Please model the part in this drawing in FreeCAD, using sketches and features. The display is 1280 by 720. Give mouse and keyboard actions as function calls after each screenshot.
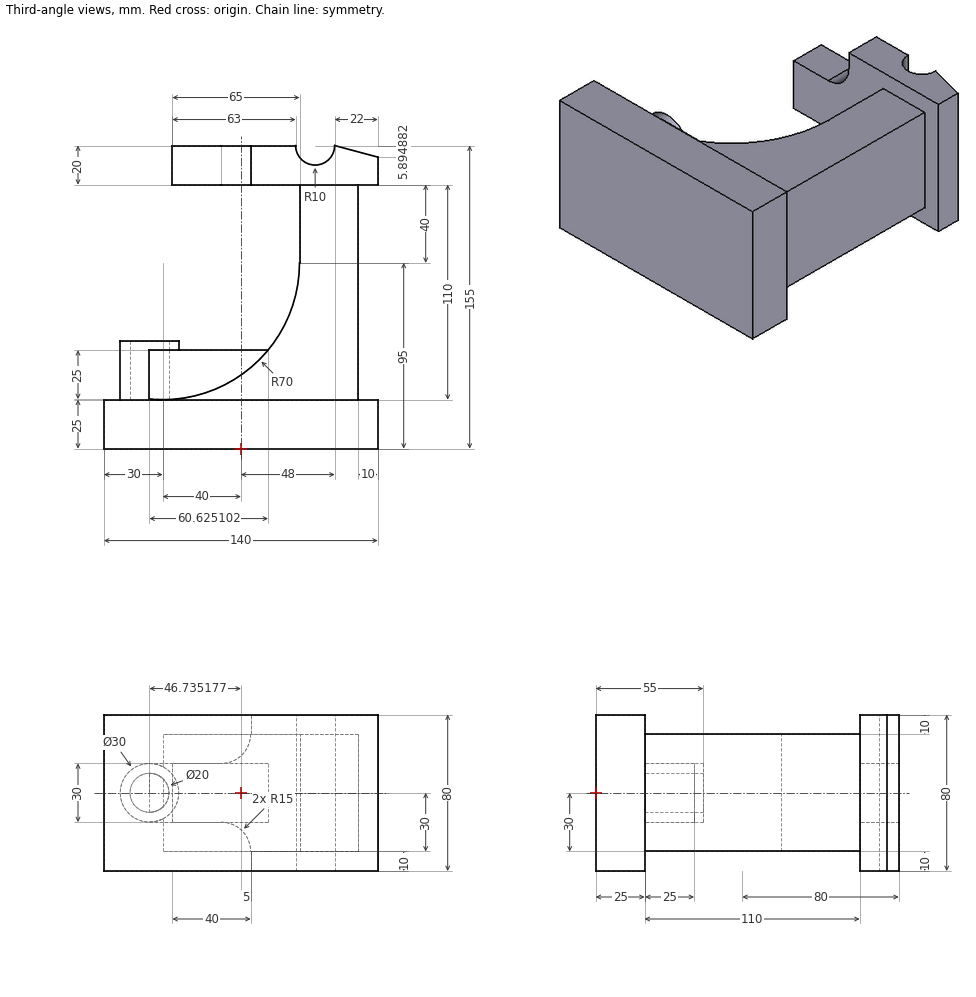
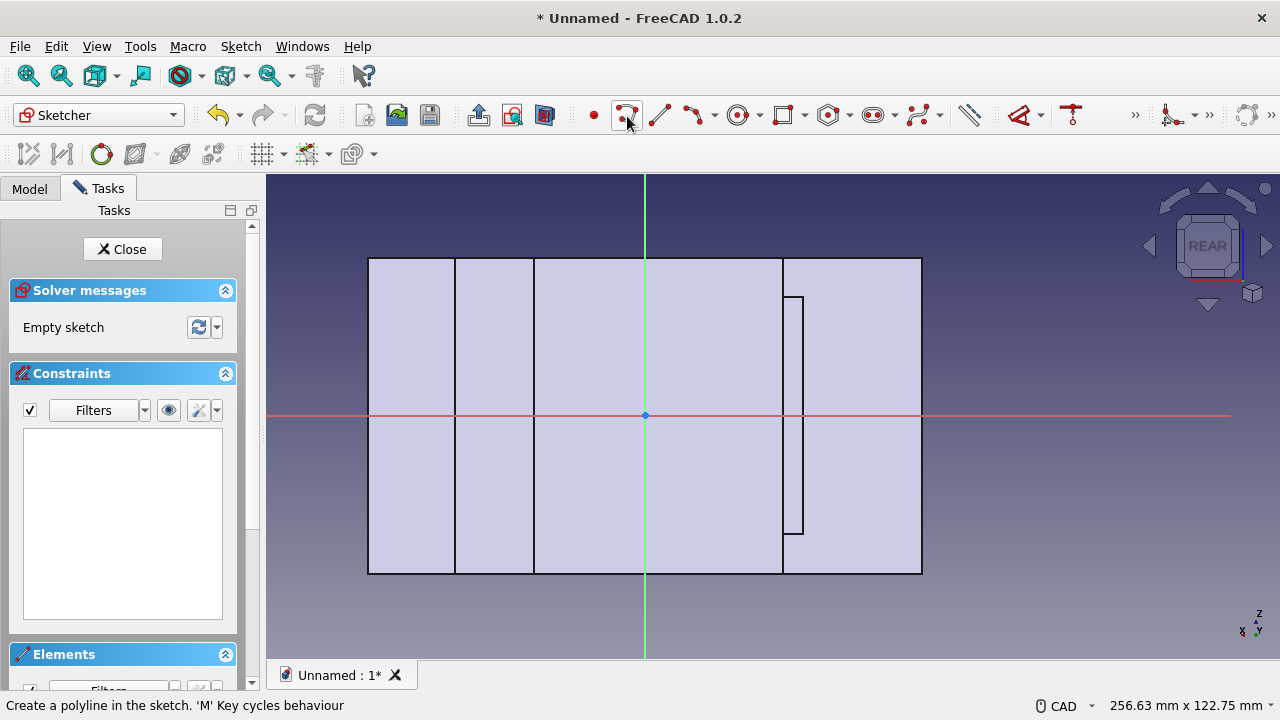
click(625, 534)
click(625, 574)
click(783, 574)
click(783, 475)
click(685, 475)
right_click(685, 475)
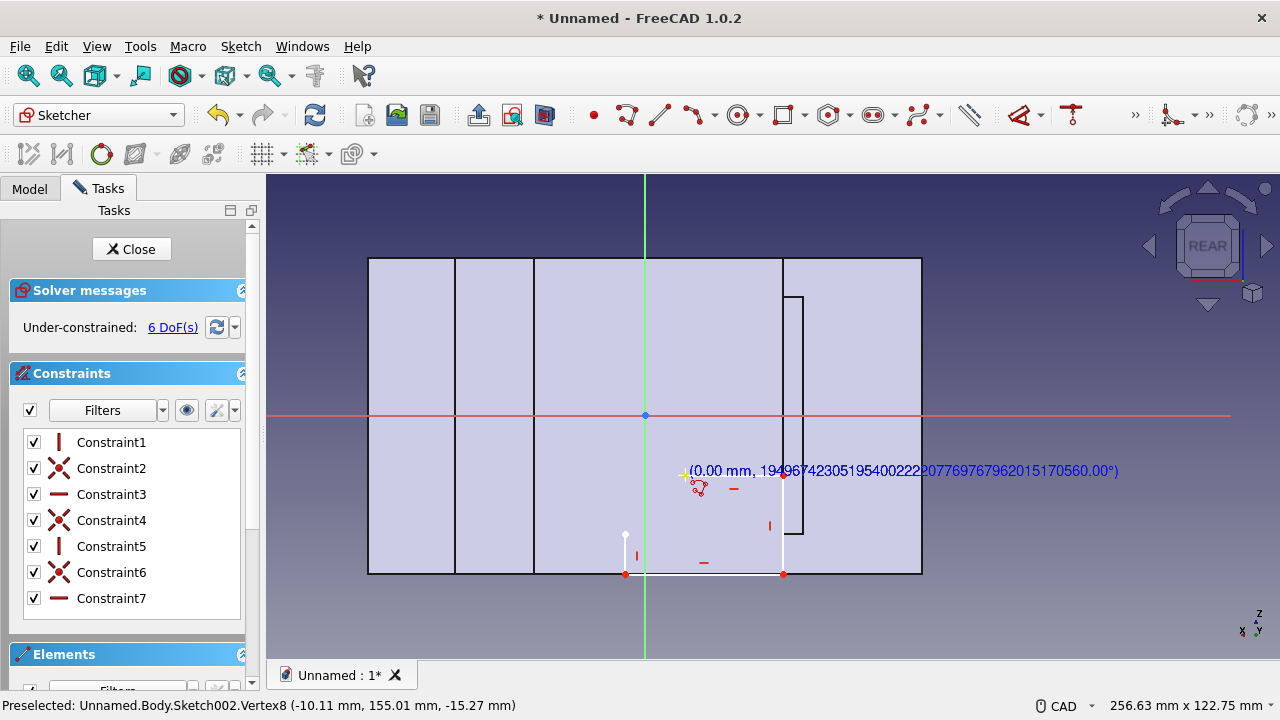
click(692, 116)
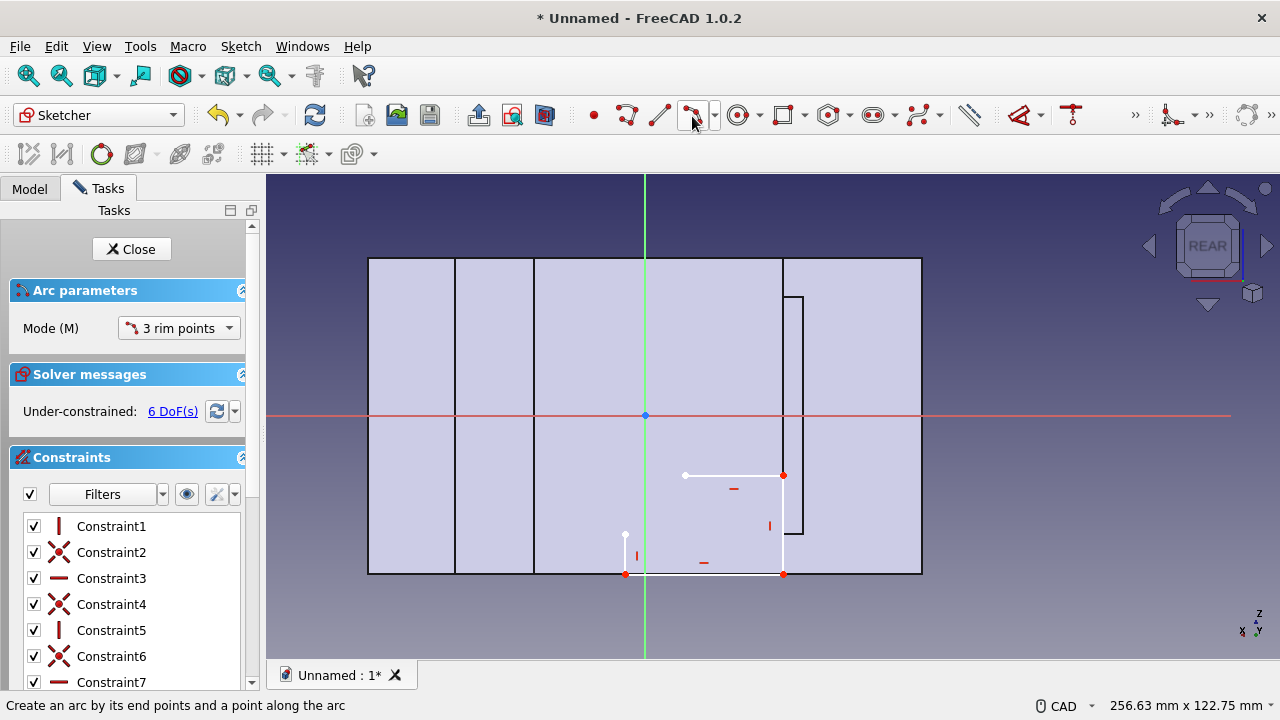
click(685, 476)
click(625, 535)
click(632, 507)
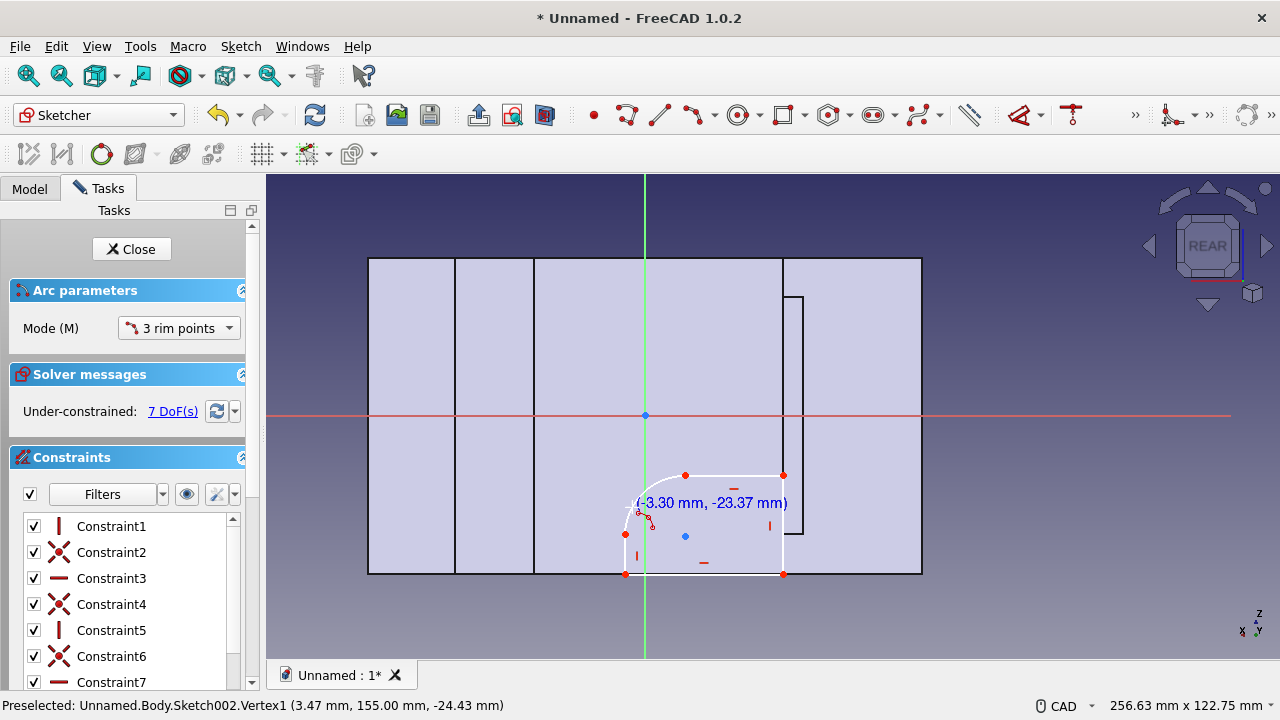
click(627, 116)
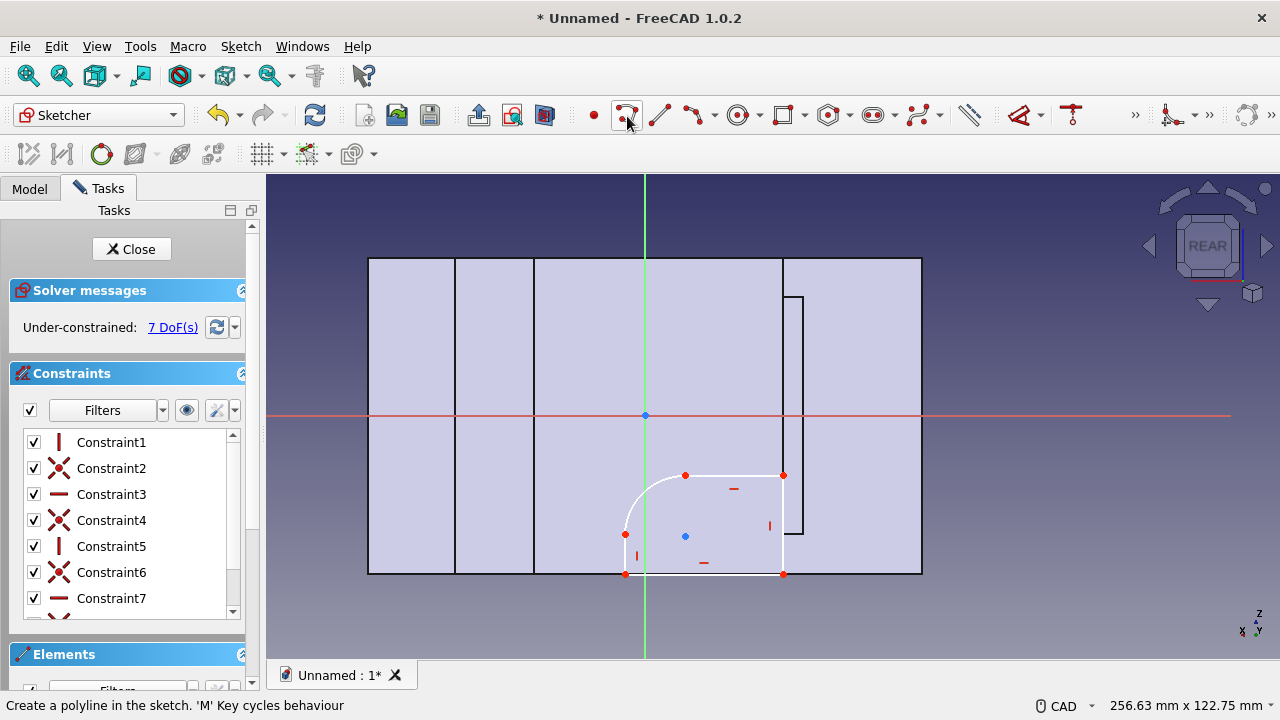
click(685, 356)
click(783, 356)
click(783, 258)
click(625, 258)
click(625, 297)
right_click(625, 297)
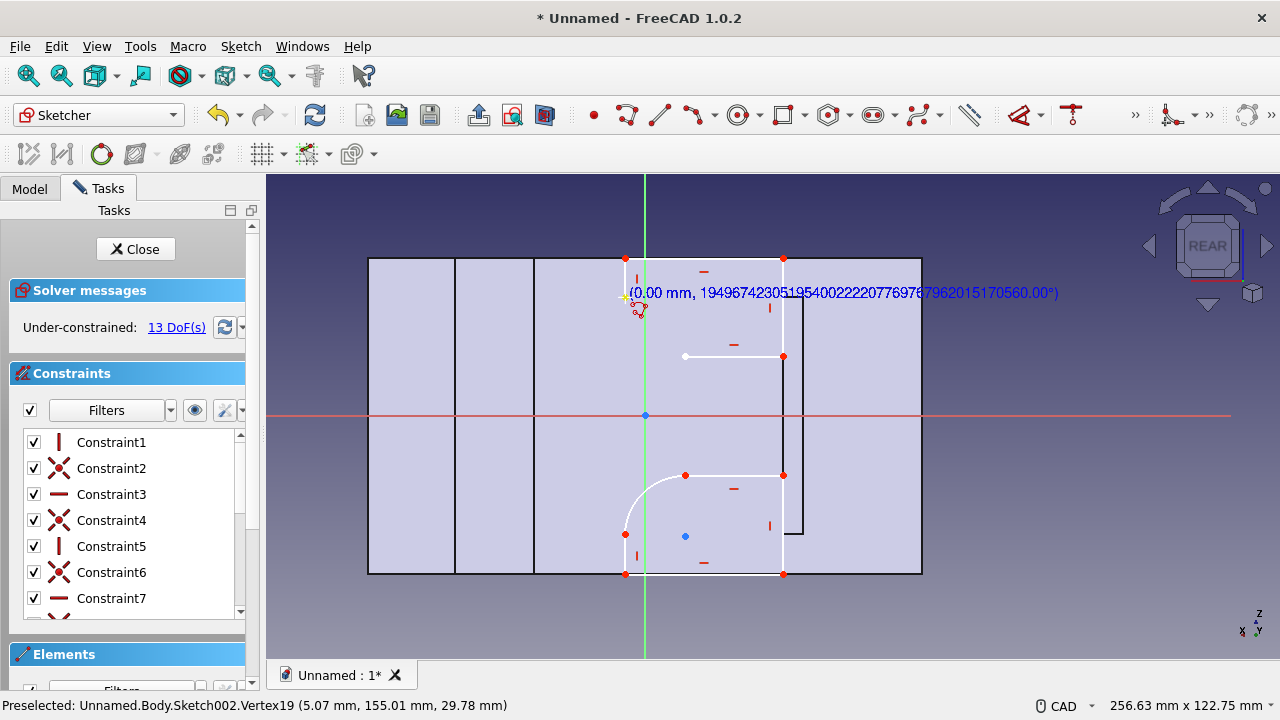
click(692, 116)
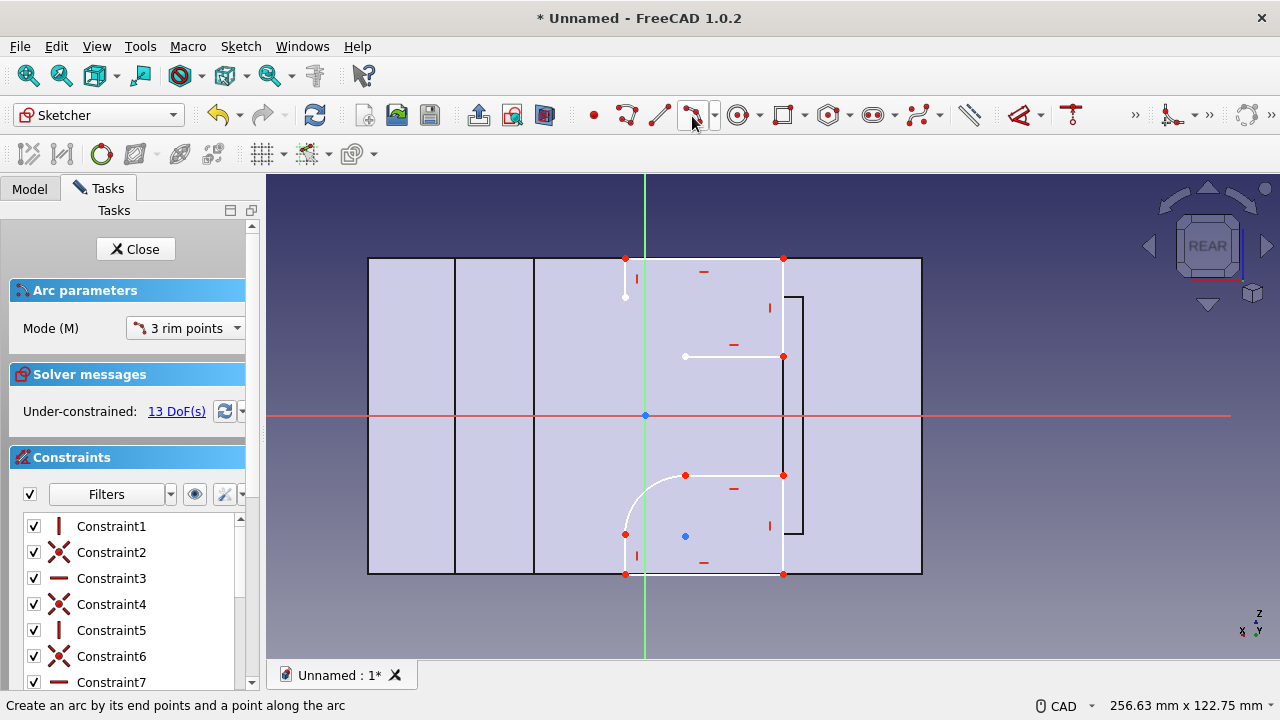
click(625, 298)
click(685, 357)
click(632, 324)
key(Escape)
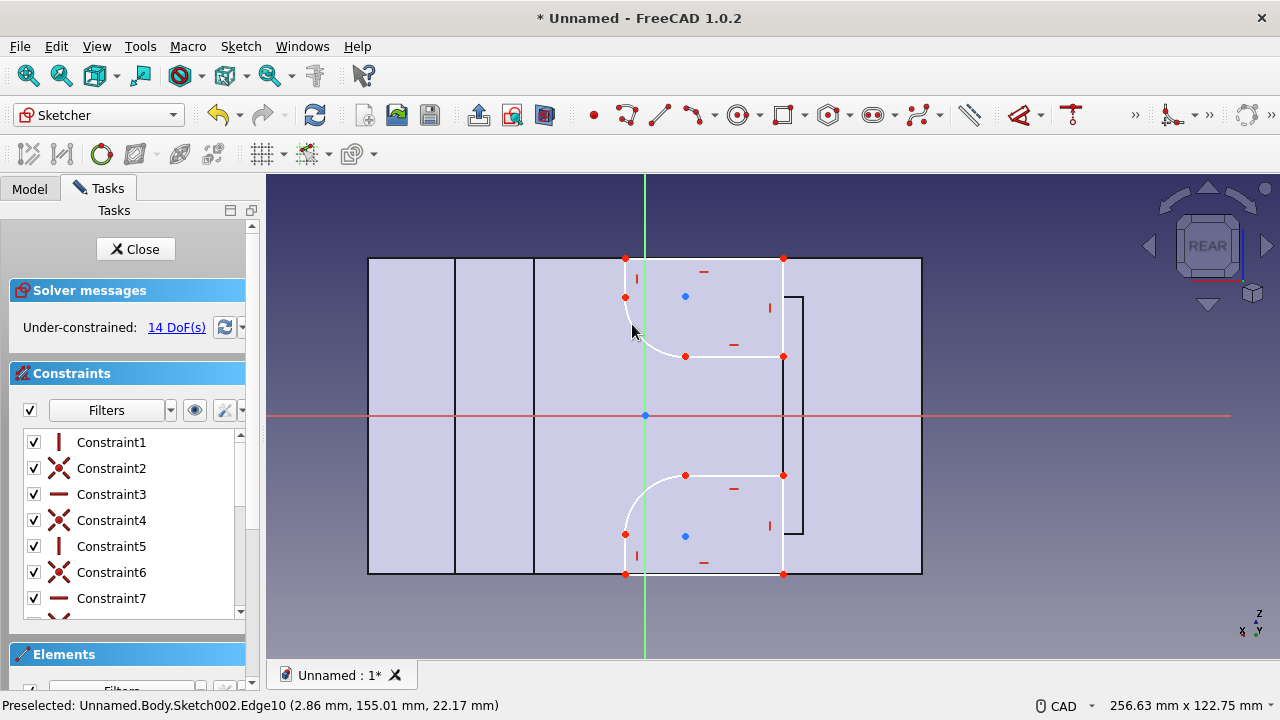
click(625, 547)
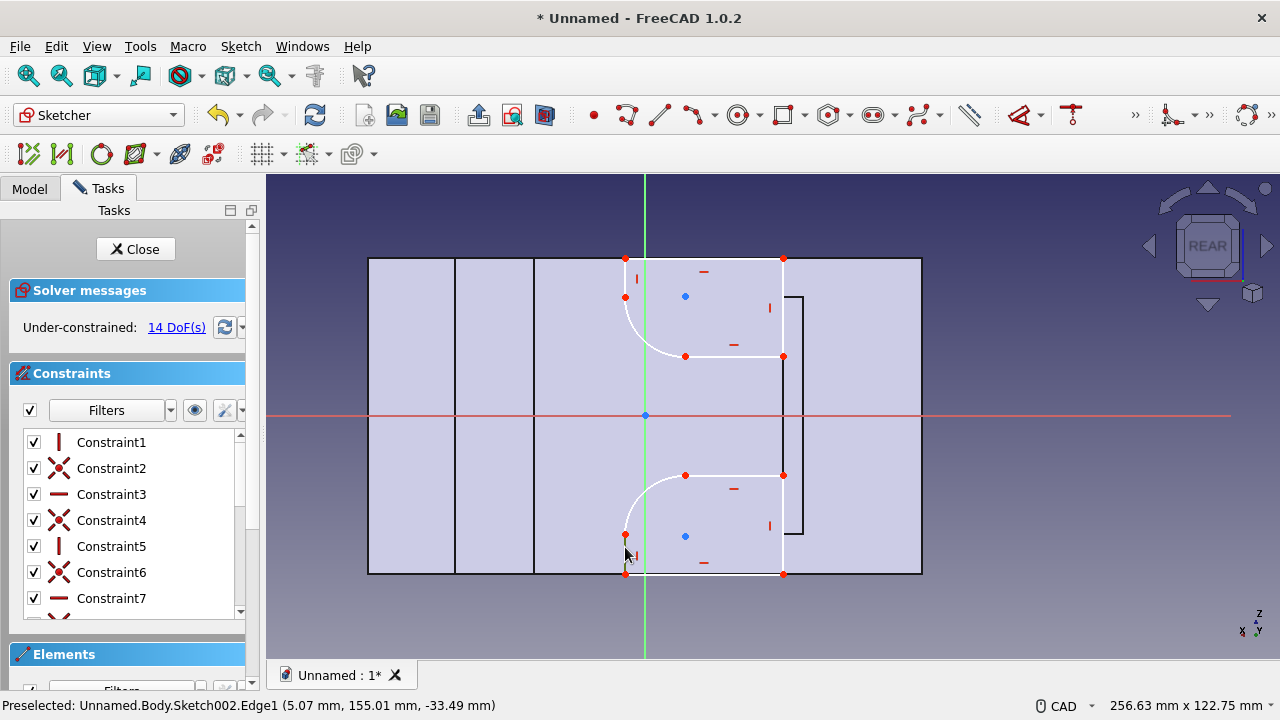
click(658, 482)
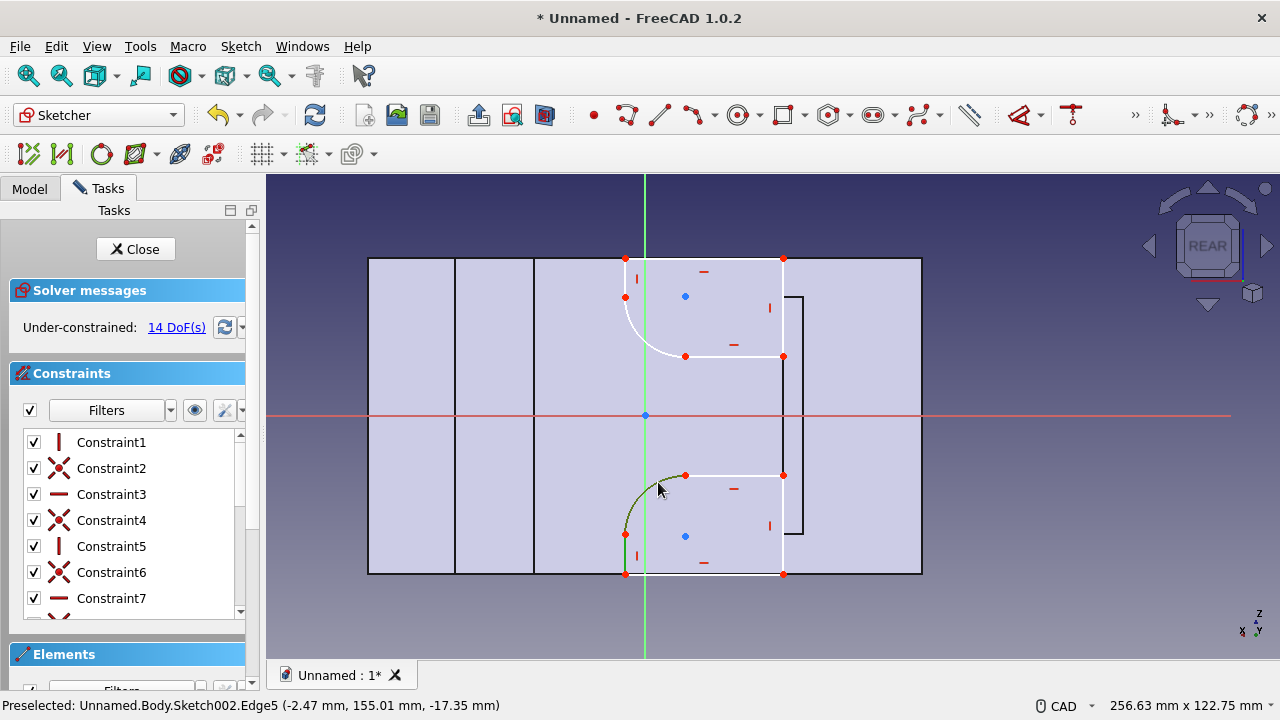
key(t)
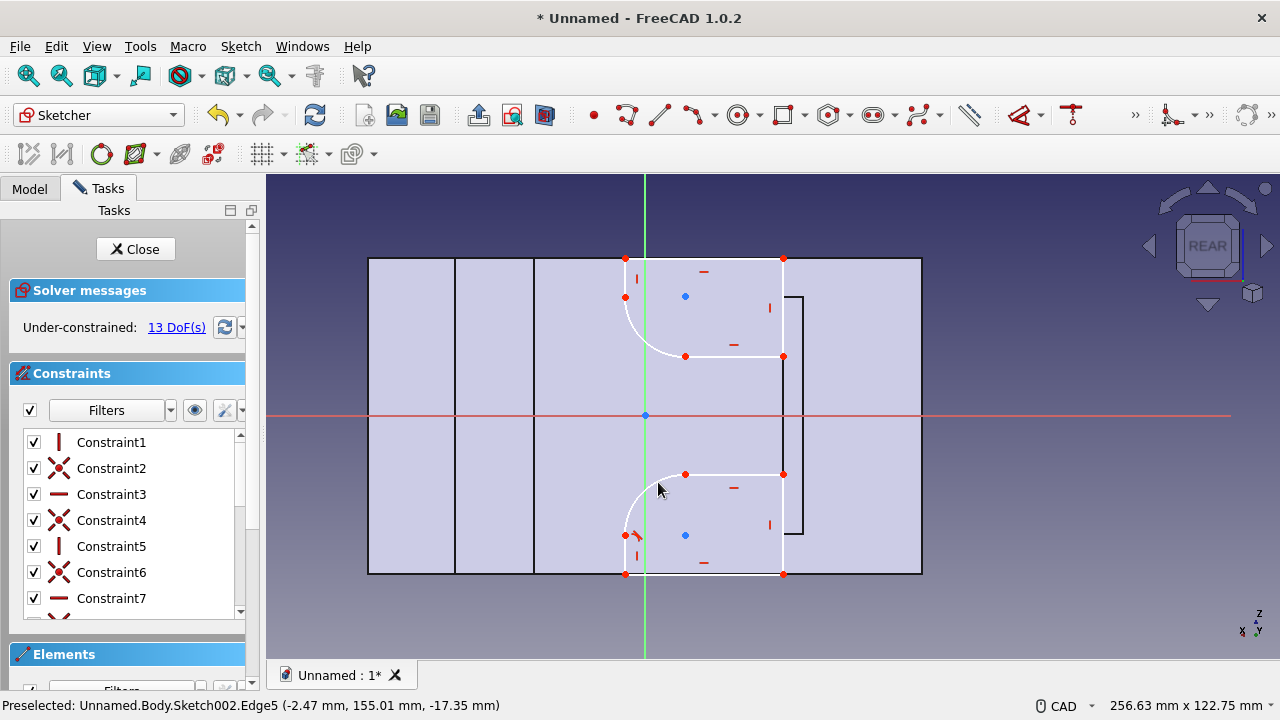
click(754, 475)